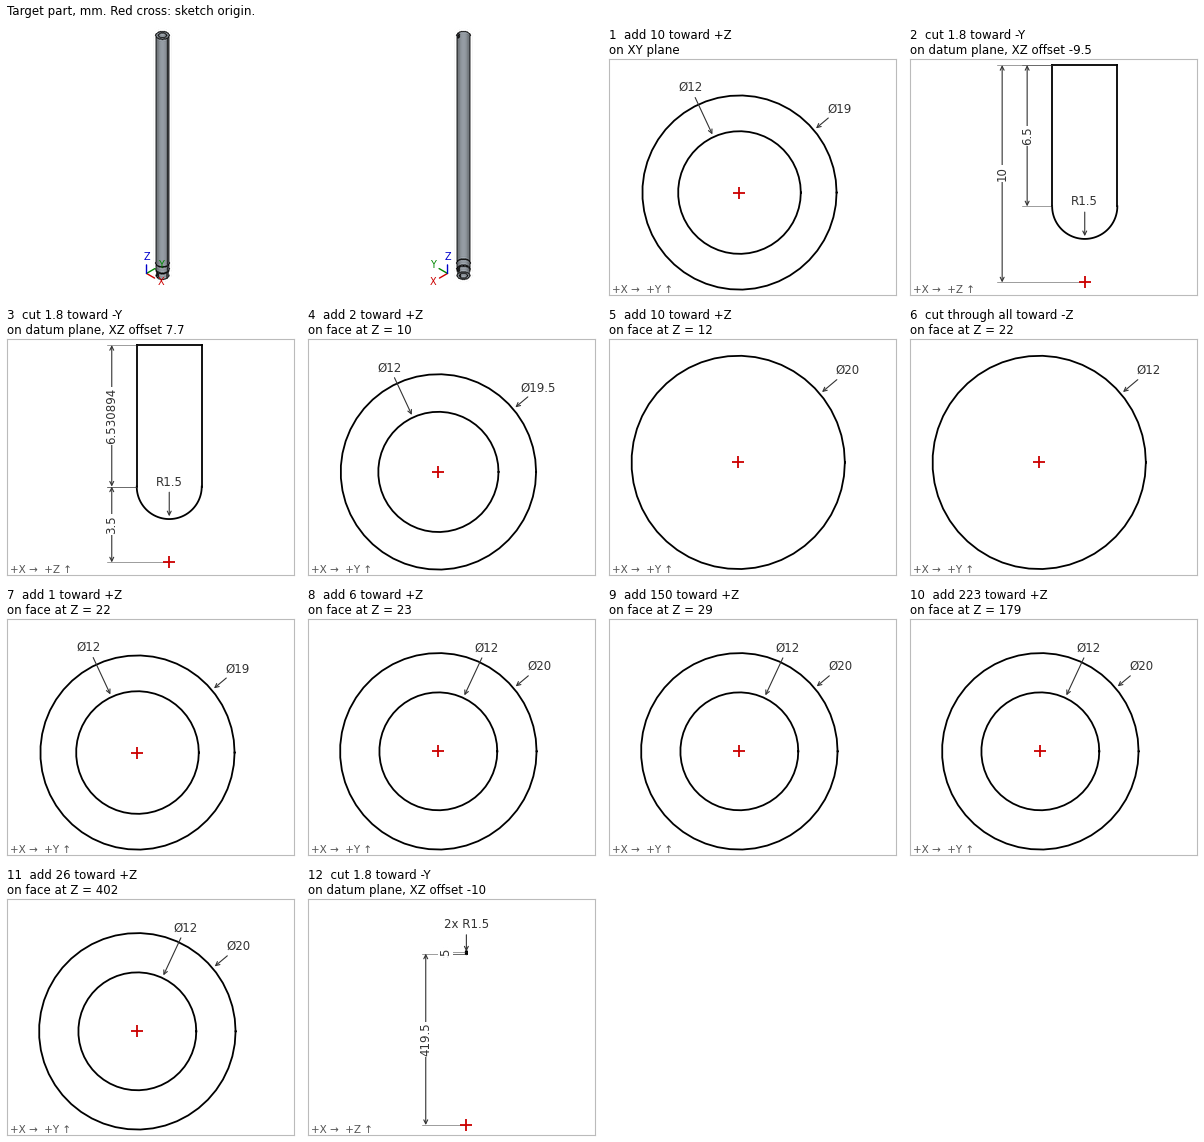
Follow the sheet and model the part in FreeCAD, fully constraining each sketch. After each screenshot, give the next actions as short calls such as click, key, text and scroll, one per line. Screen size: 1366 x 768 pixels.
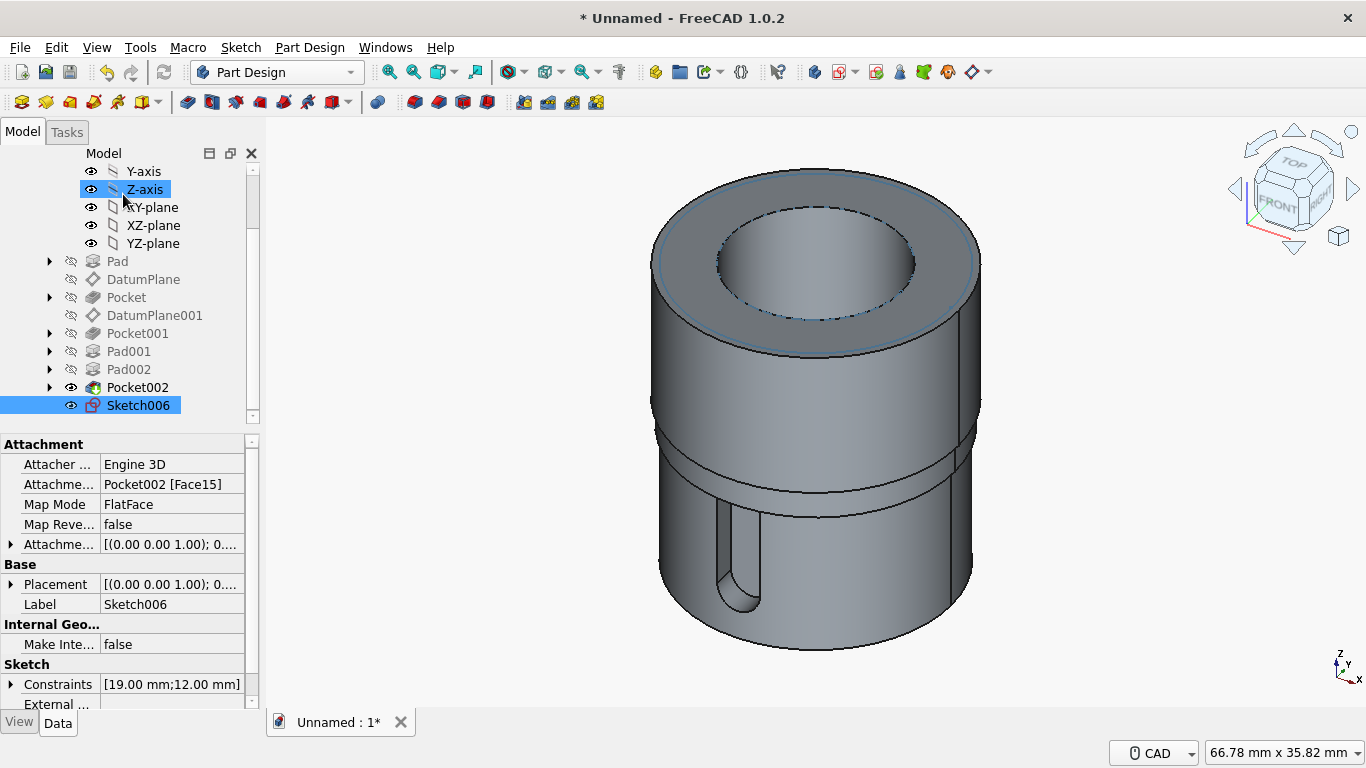
click(22, 102)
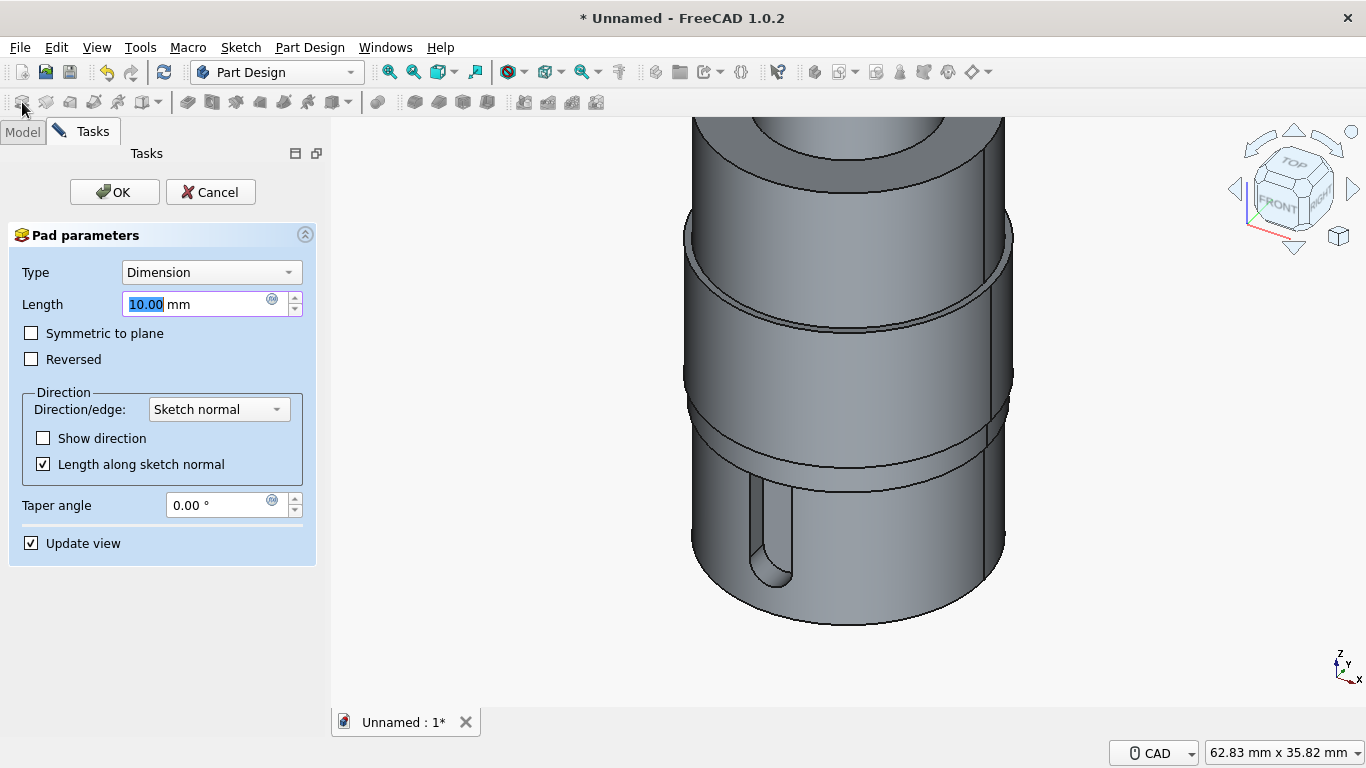
text(1)
key(Tab)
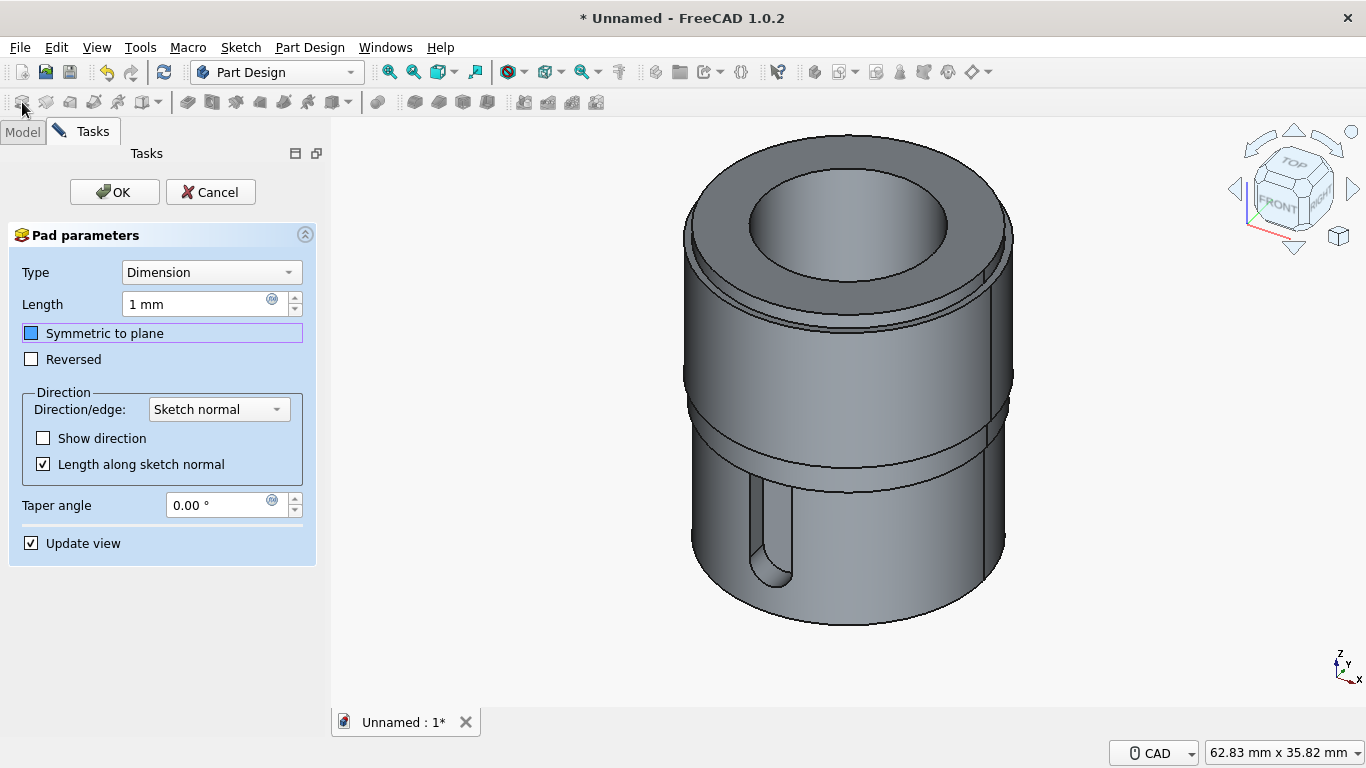
click(115, 192)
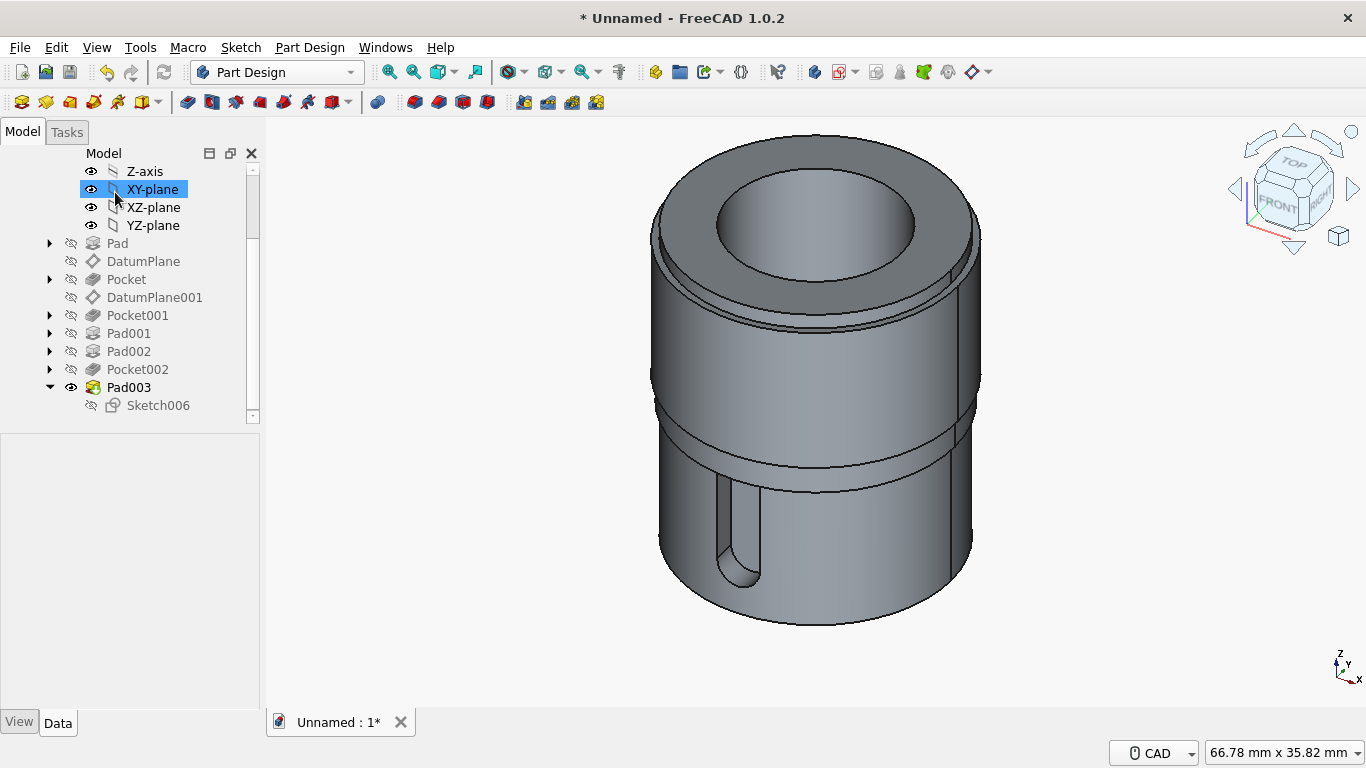
click(390, 72)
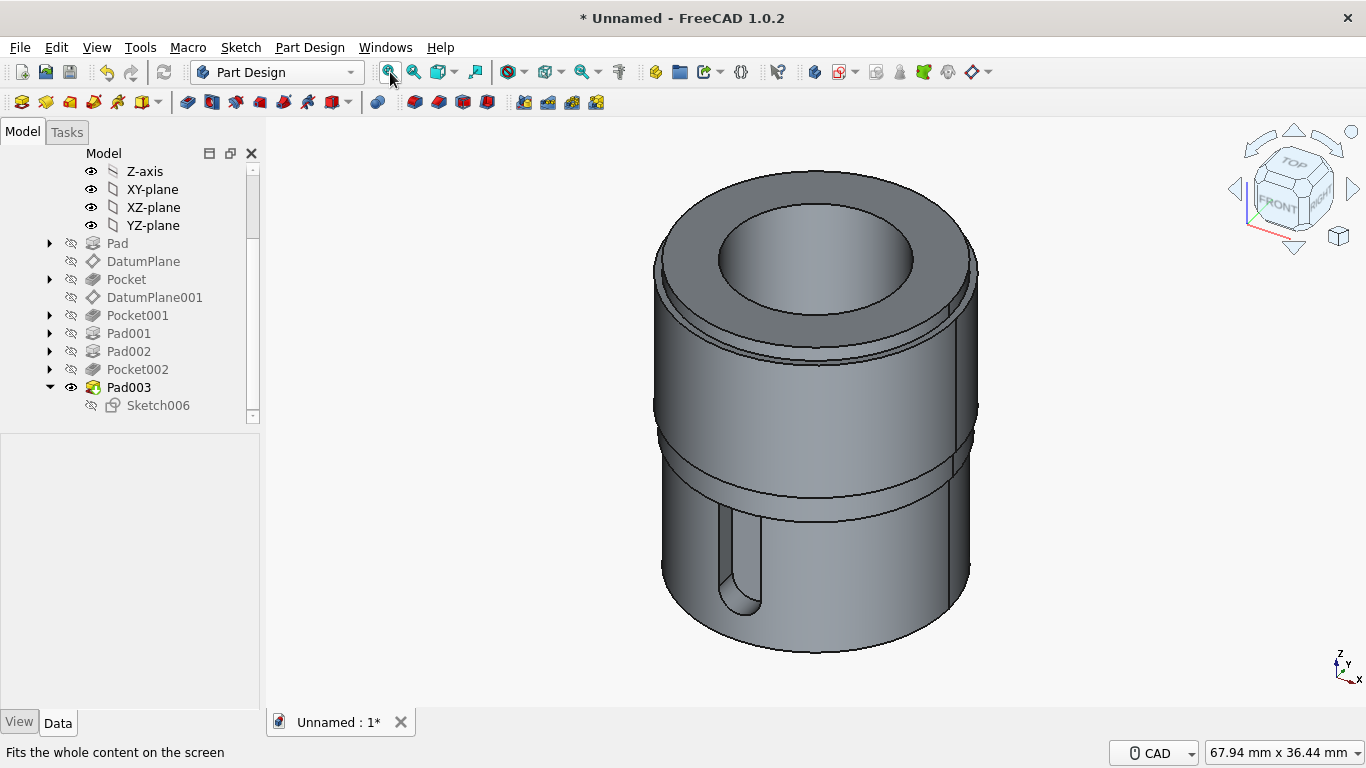
click(784, 190)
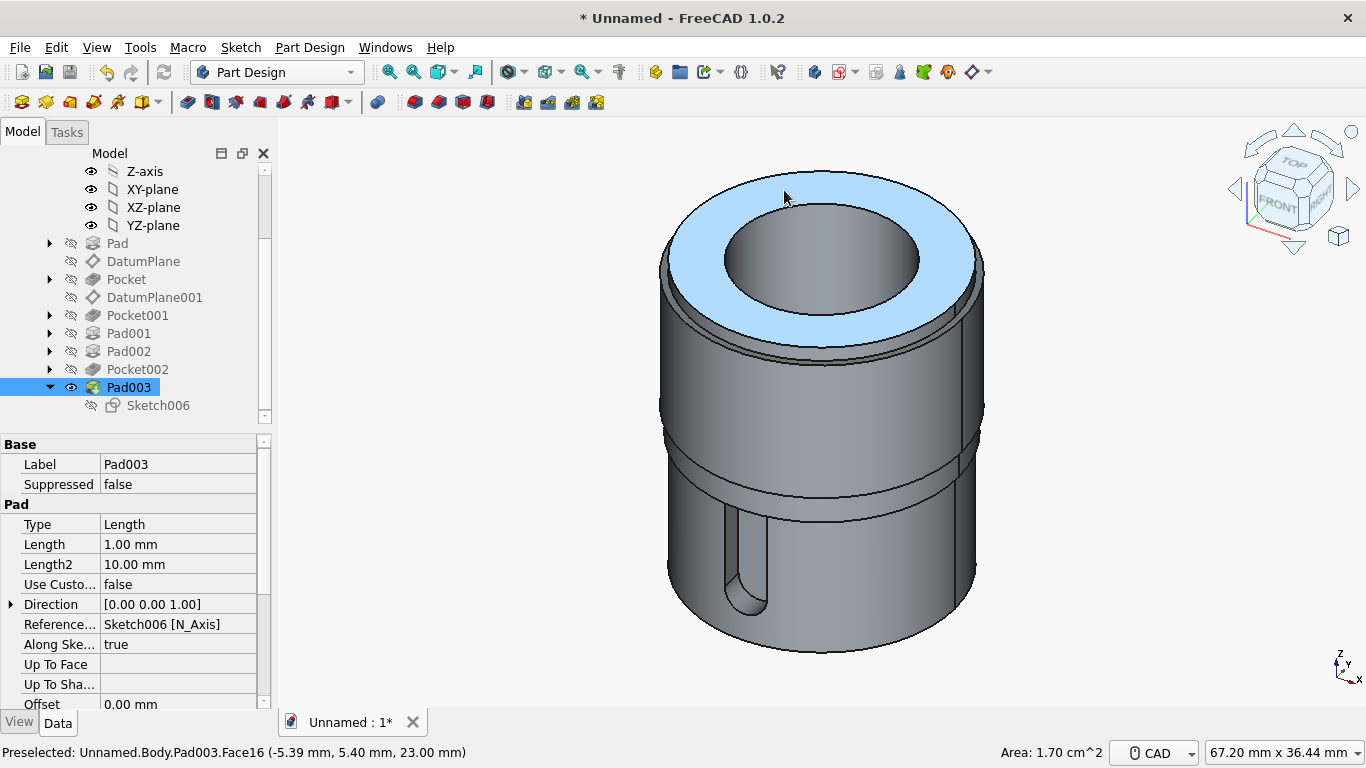
click(840, 72)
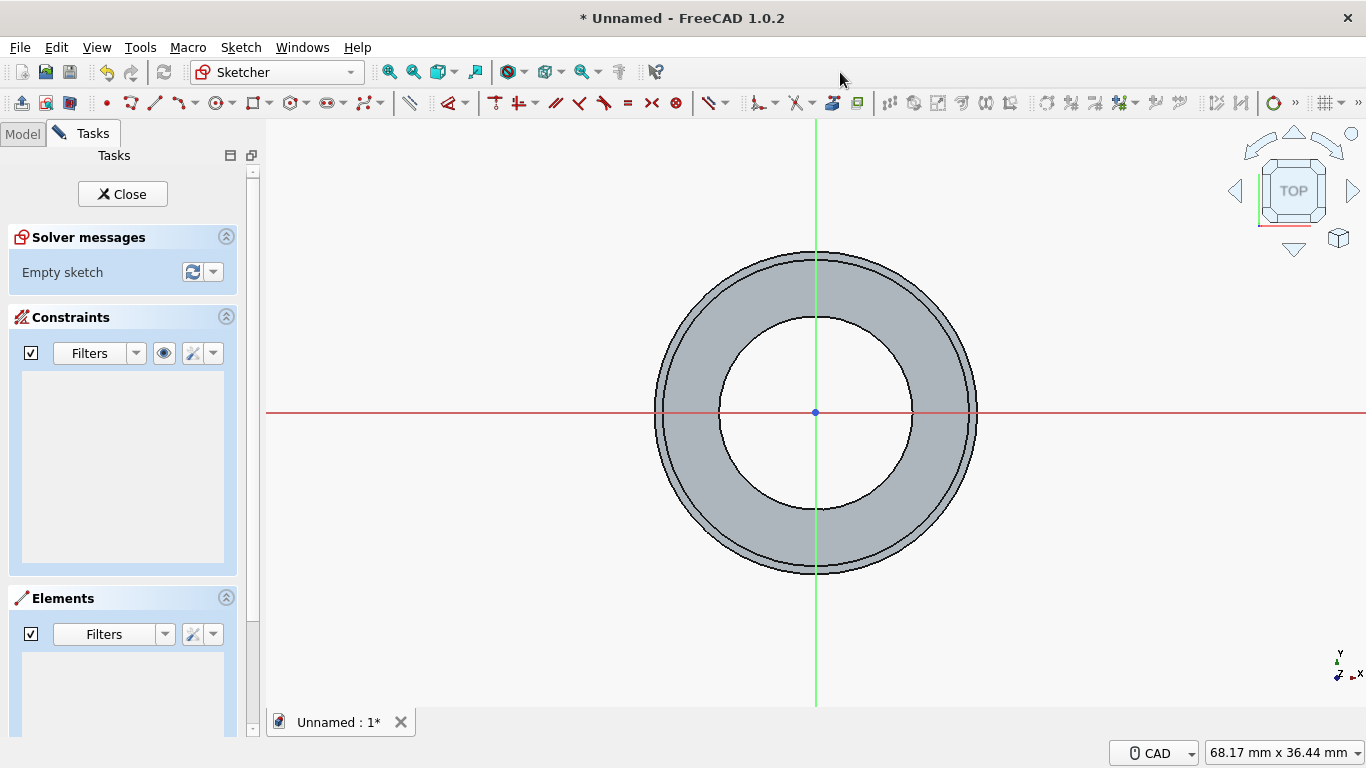
click(216, 104)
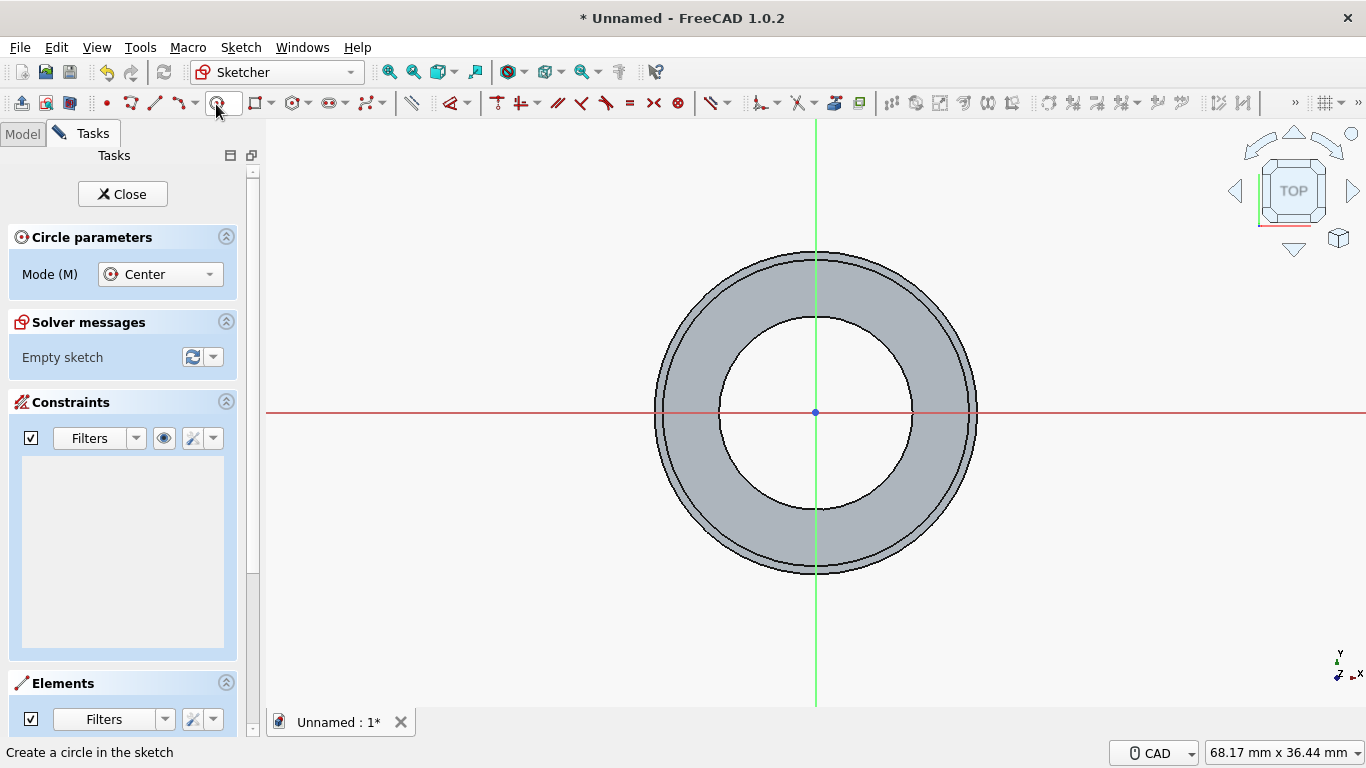
click(816, 413)
click(930, 299)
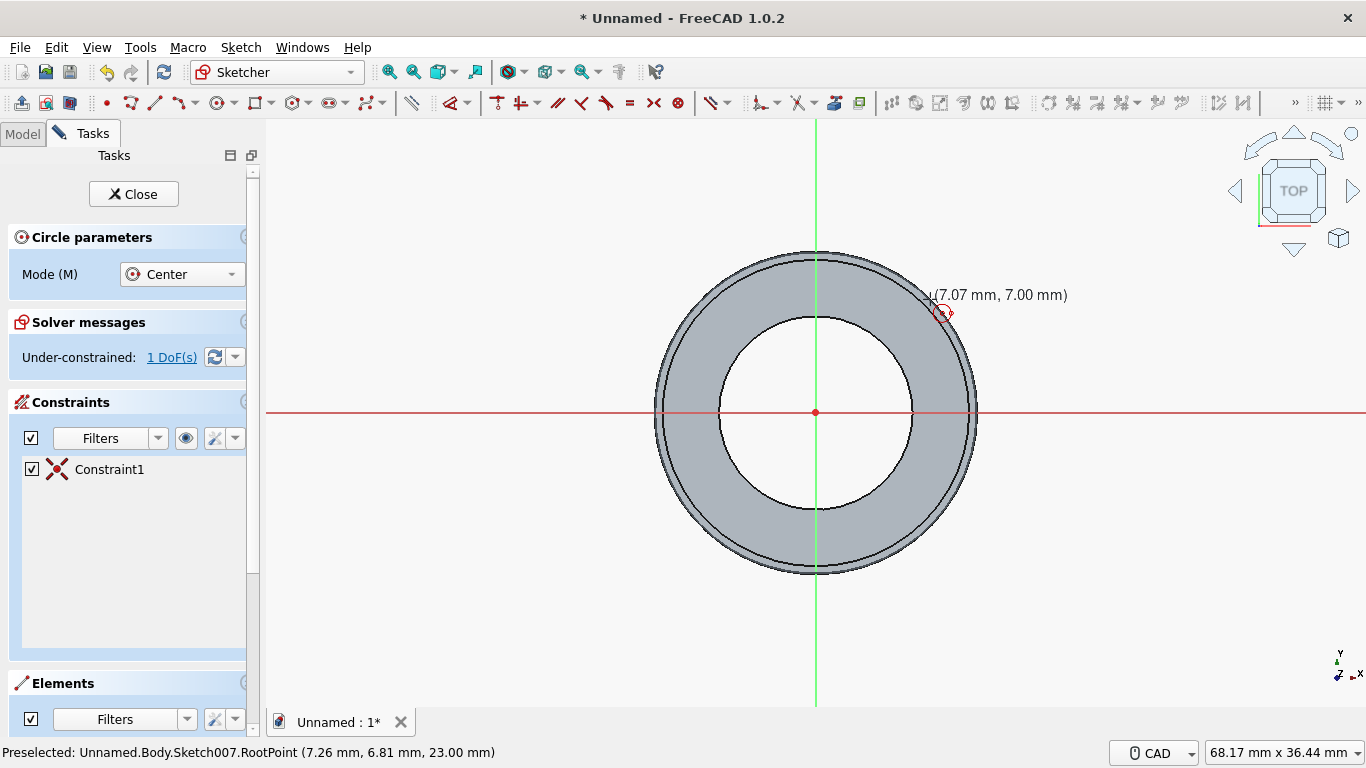
click(816, 413)
click(884, 345)
key(Escape)